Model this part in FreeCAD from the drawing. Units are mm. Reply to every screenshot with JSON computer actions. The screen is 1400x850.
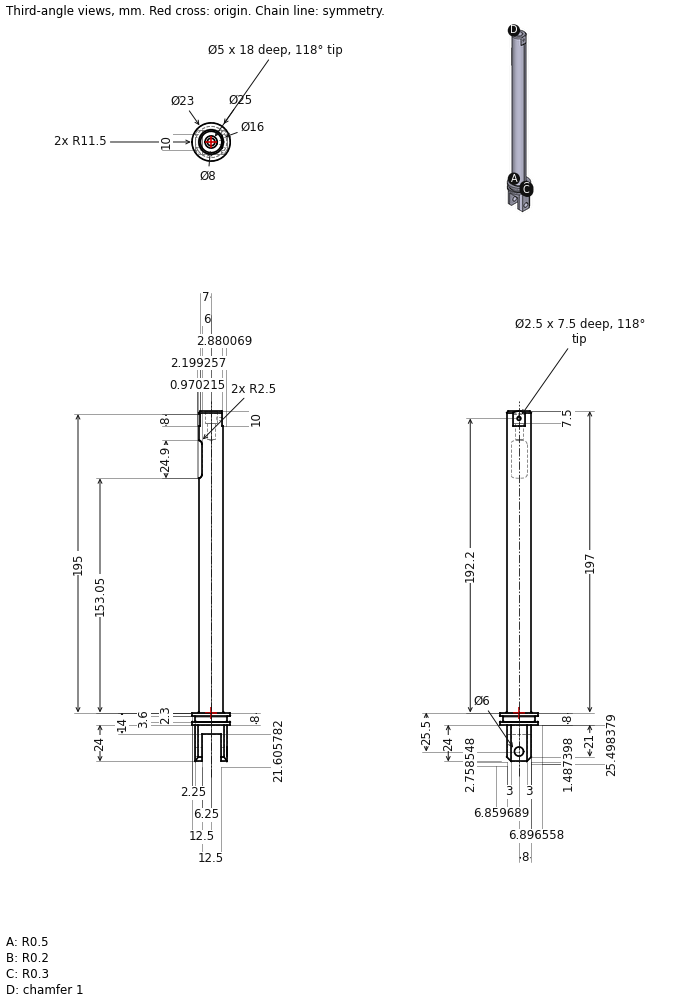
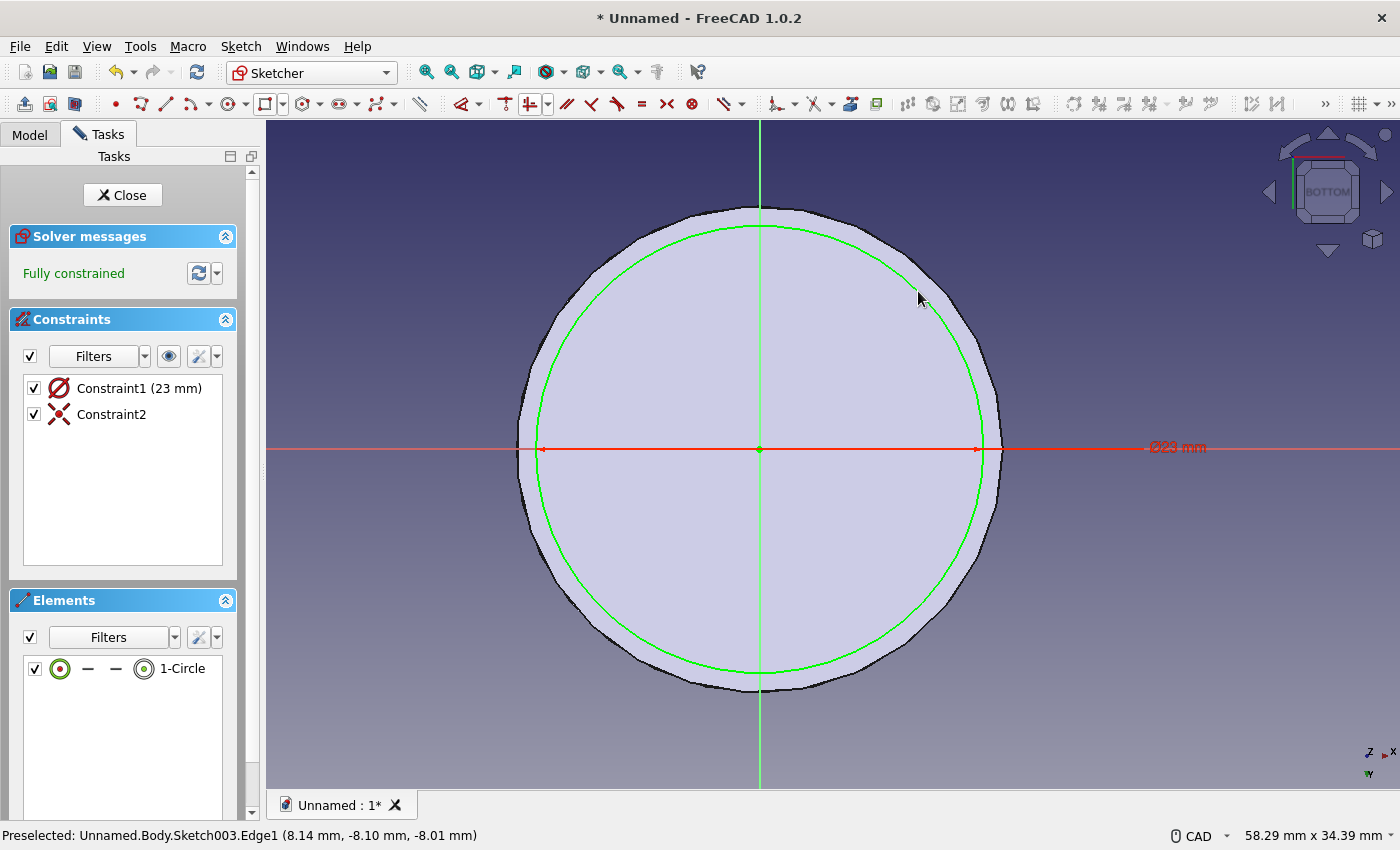
{"action": "left_click", "coordinate": [123, 195]}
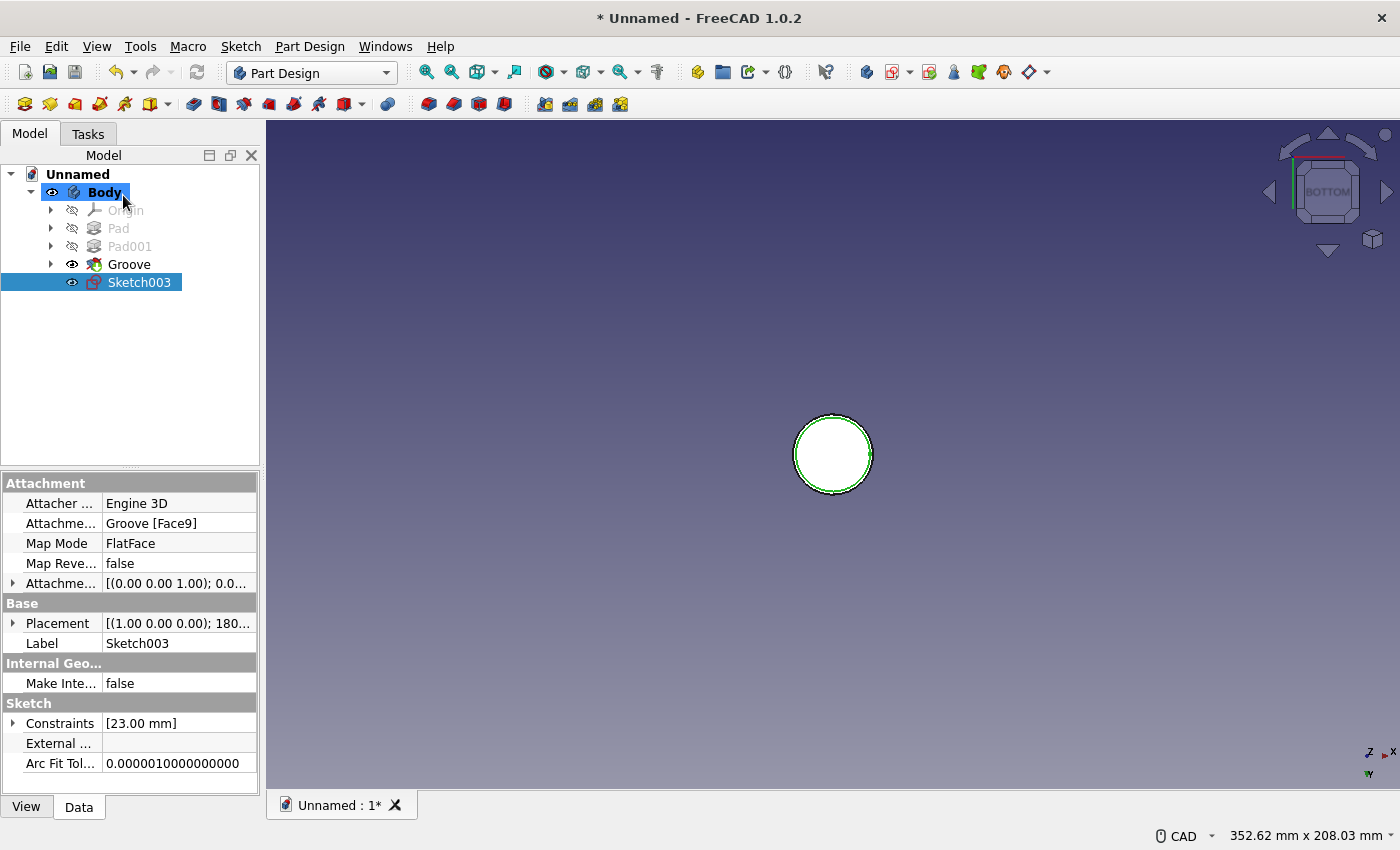
{"action": "left_click", "coordinate": [25, 104]}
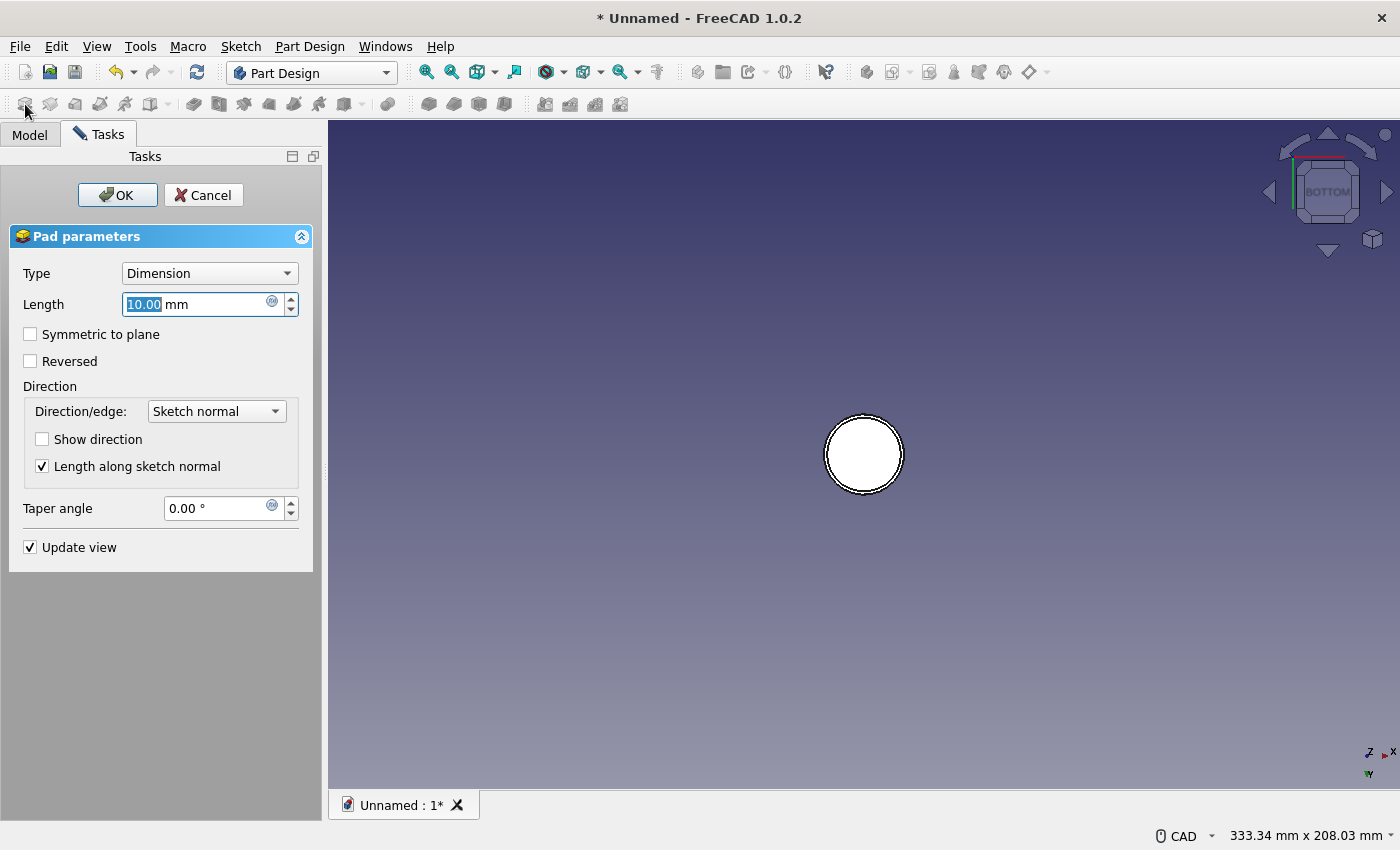
{"action": "type", "text": "24"}
{"action": "key", "text": "Tab"}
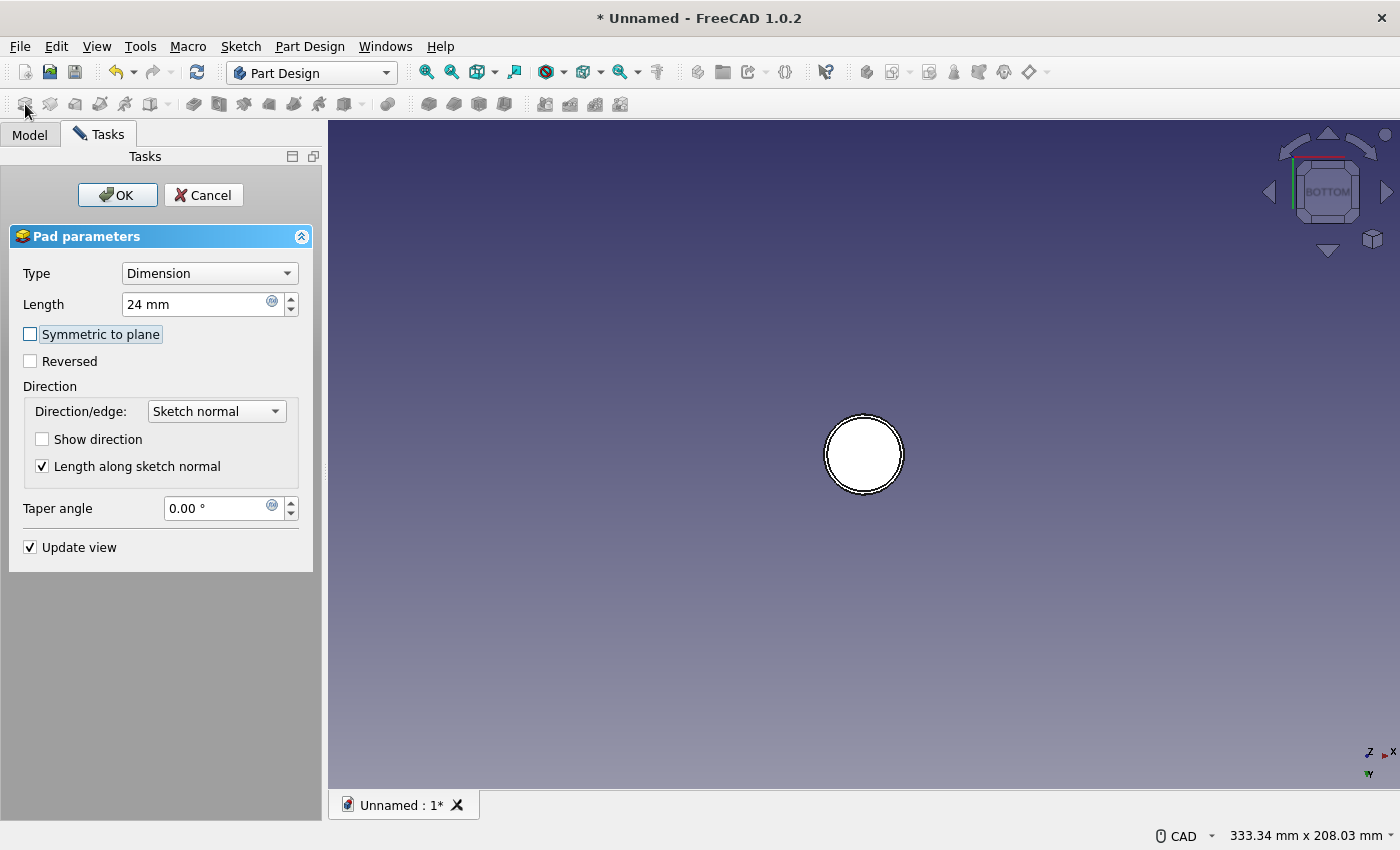
{"action": "left_click", "coordinate": [118, 195]}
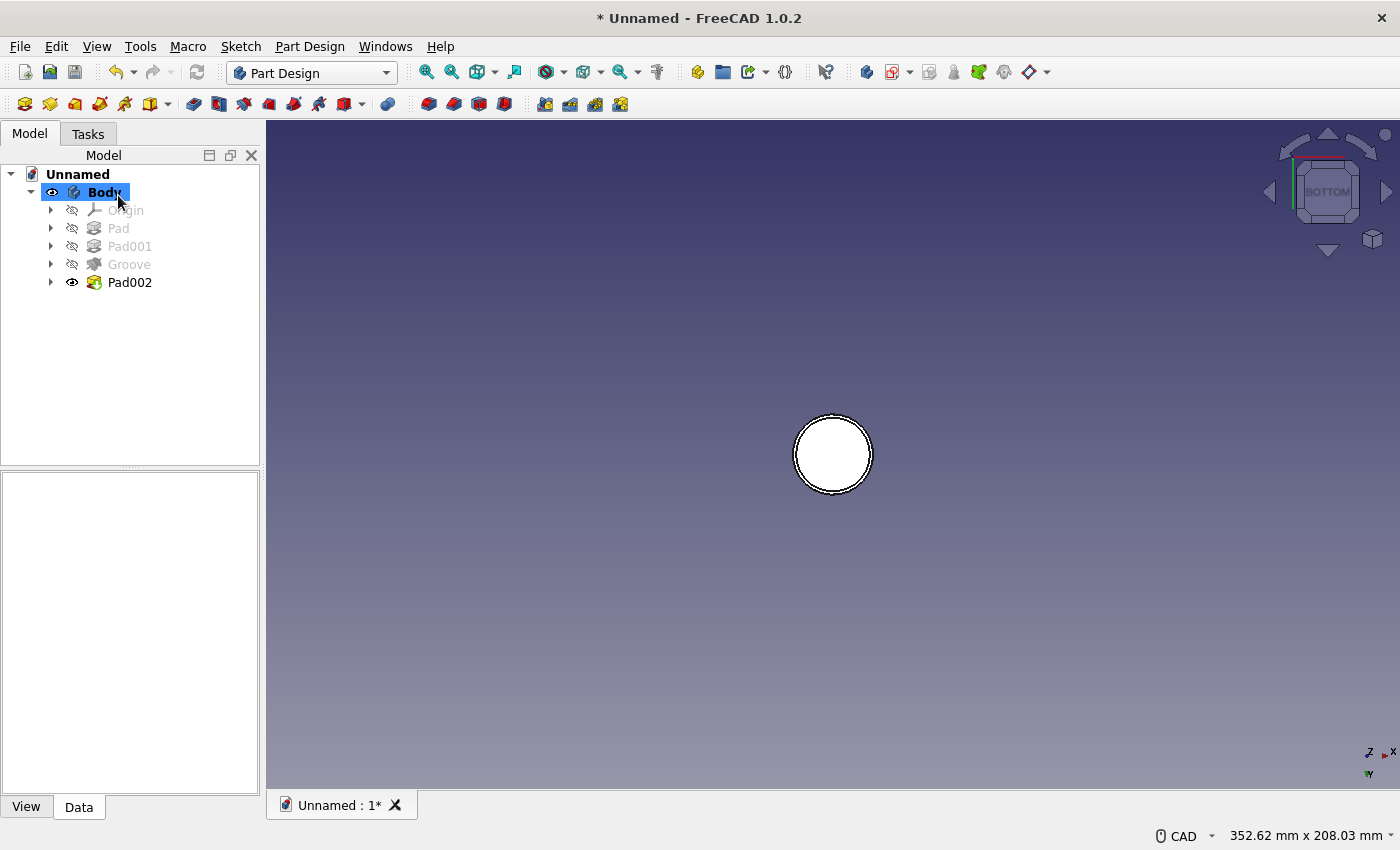
{"action": "left_click", "coordinate": [427, 72]}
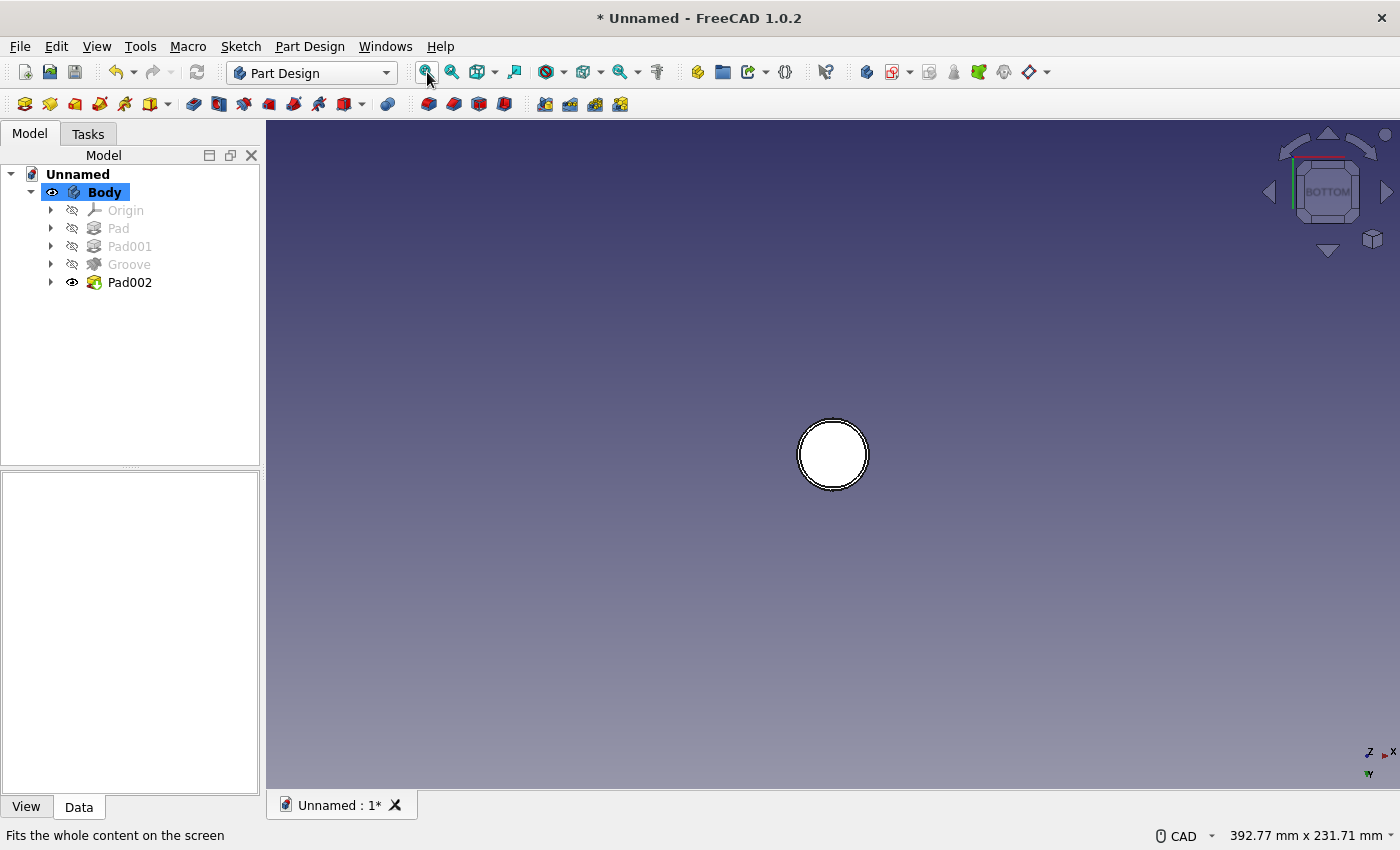
{"action": "left_click", "coordinate": [892, 72]}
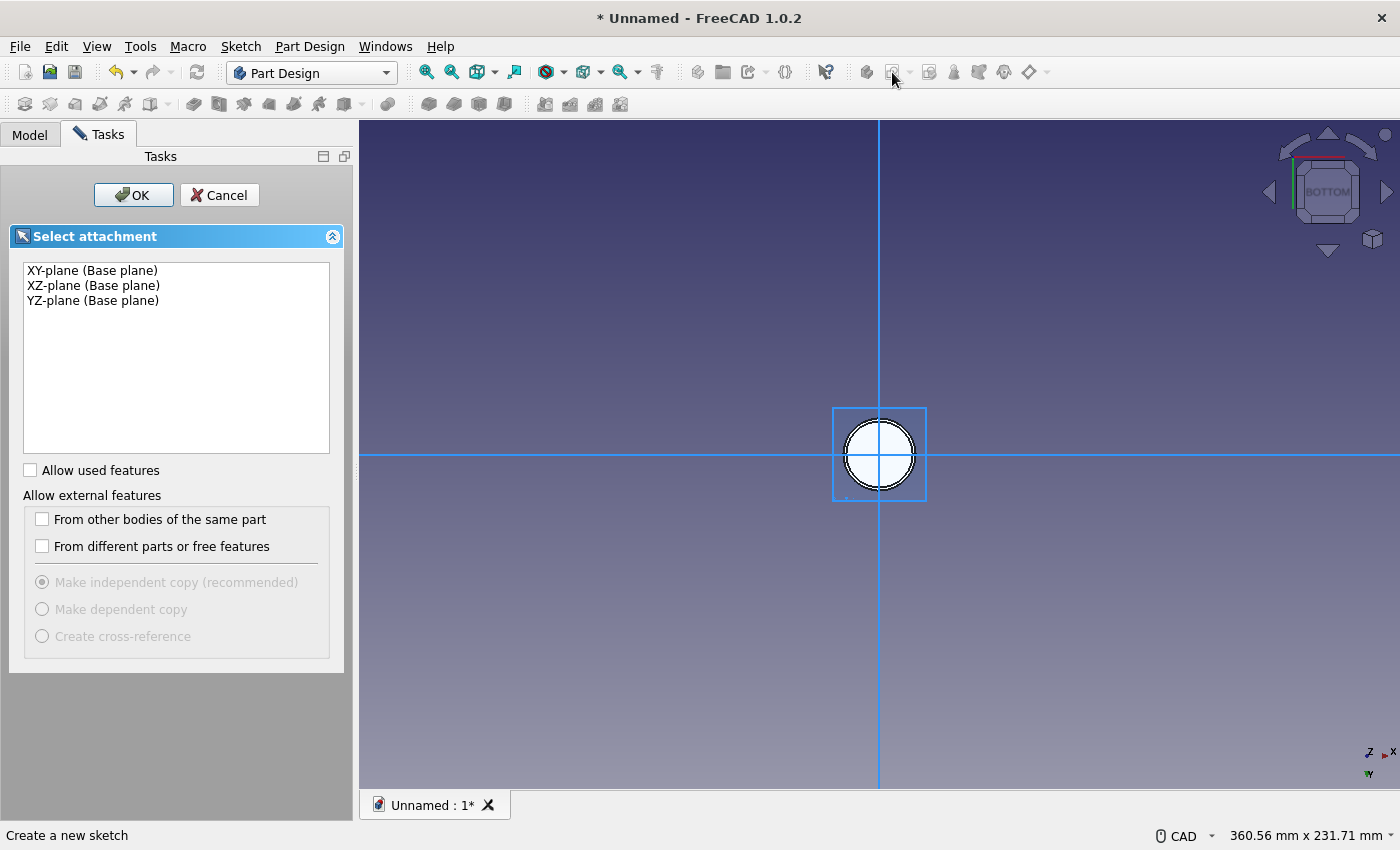
{"action": "left_click", "coordinate": [84, 286]}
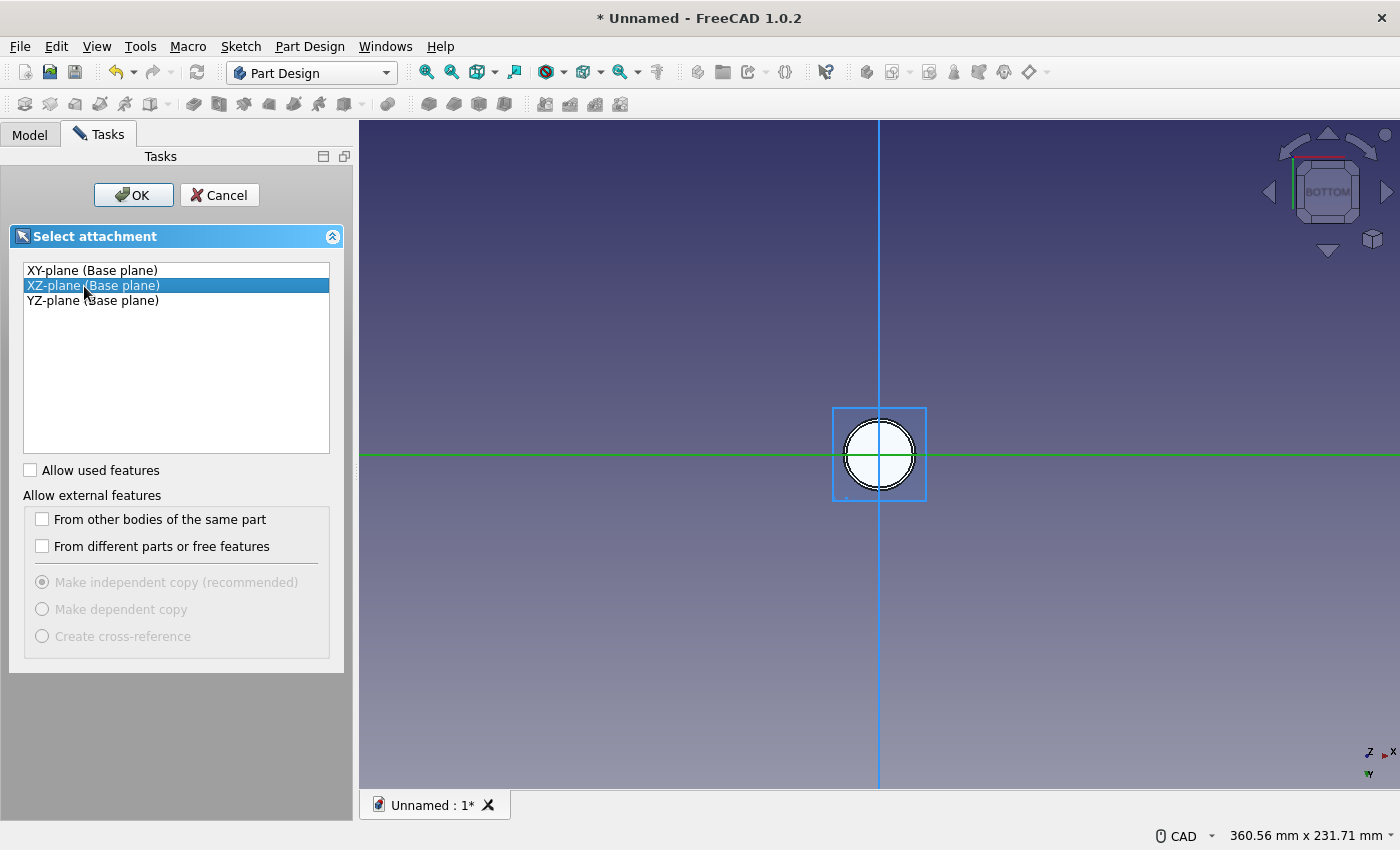
{"action": "left_click", "coordinate": [134, 195]}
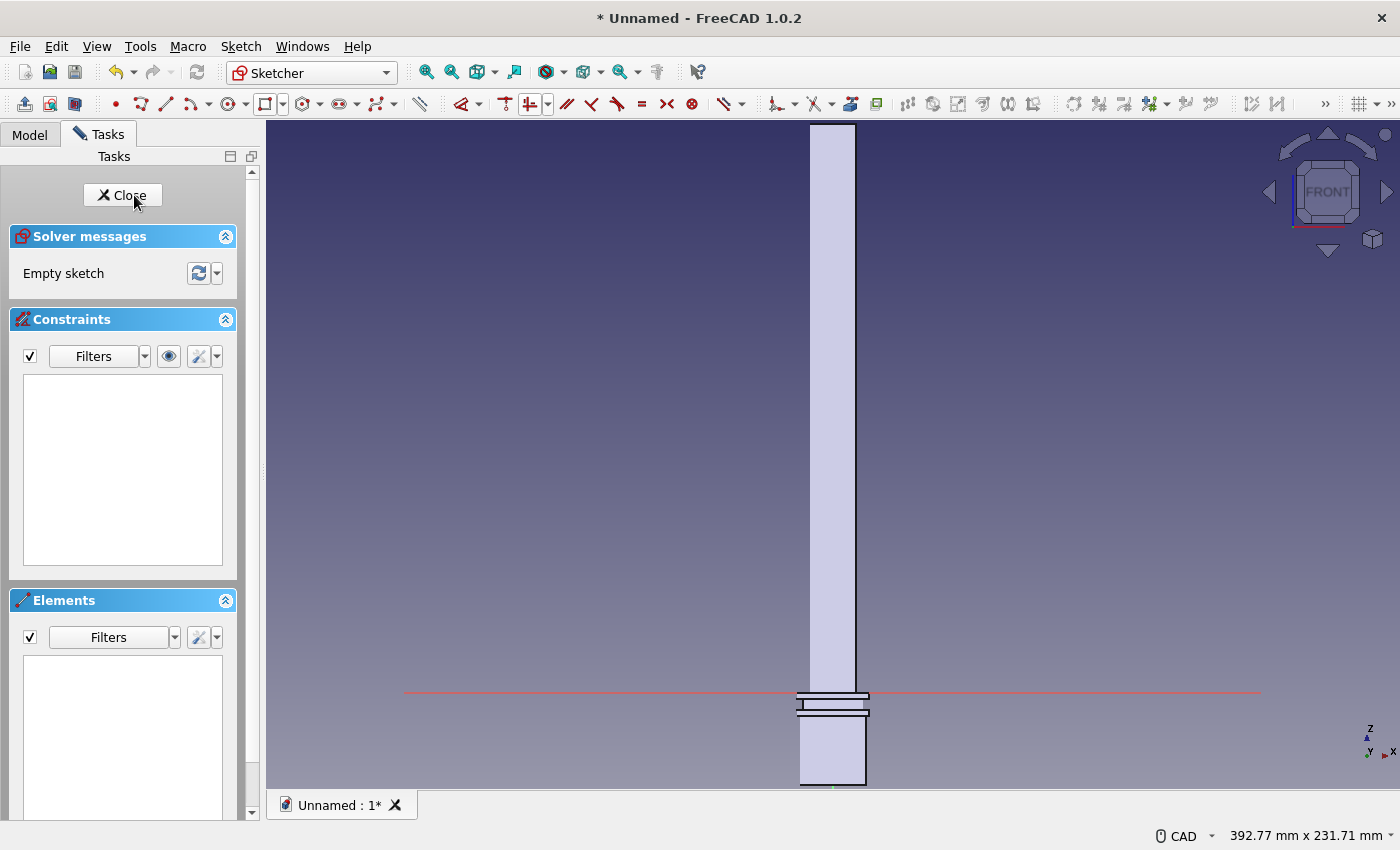
{"action": "left_click", "coordinate": [75, 104]}